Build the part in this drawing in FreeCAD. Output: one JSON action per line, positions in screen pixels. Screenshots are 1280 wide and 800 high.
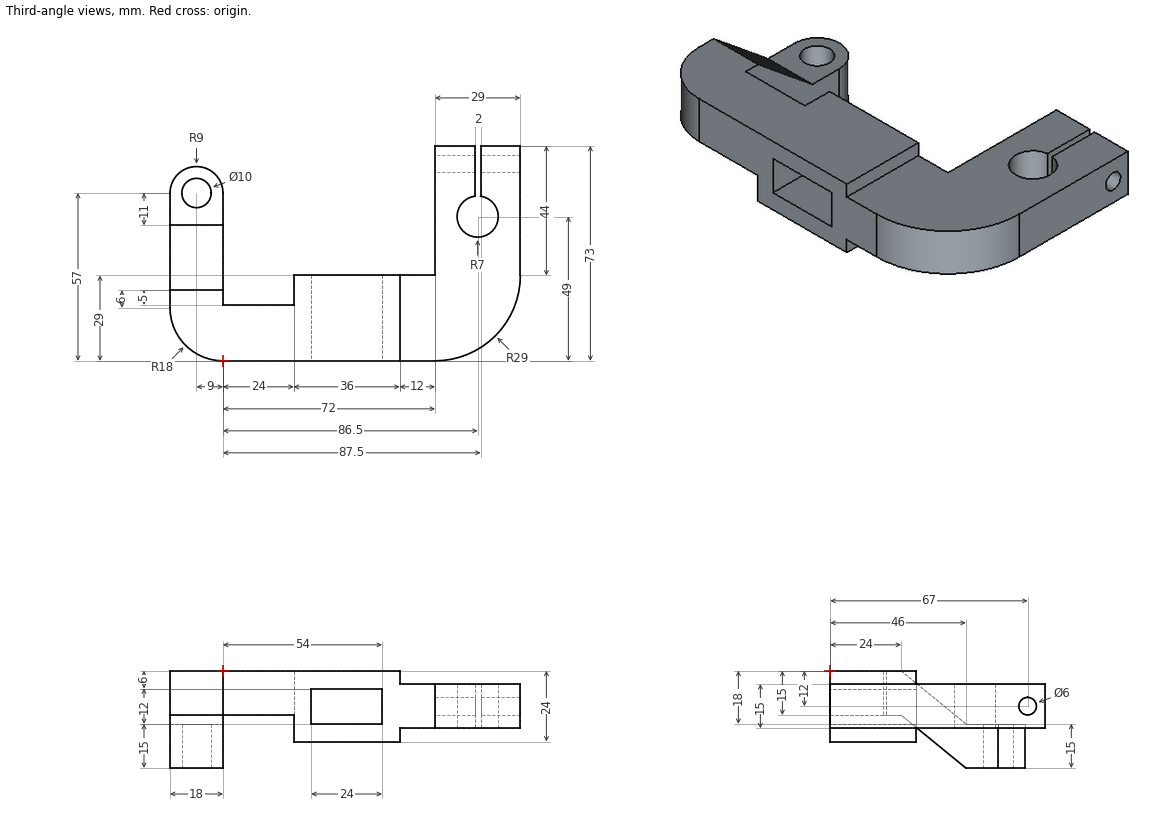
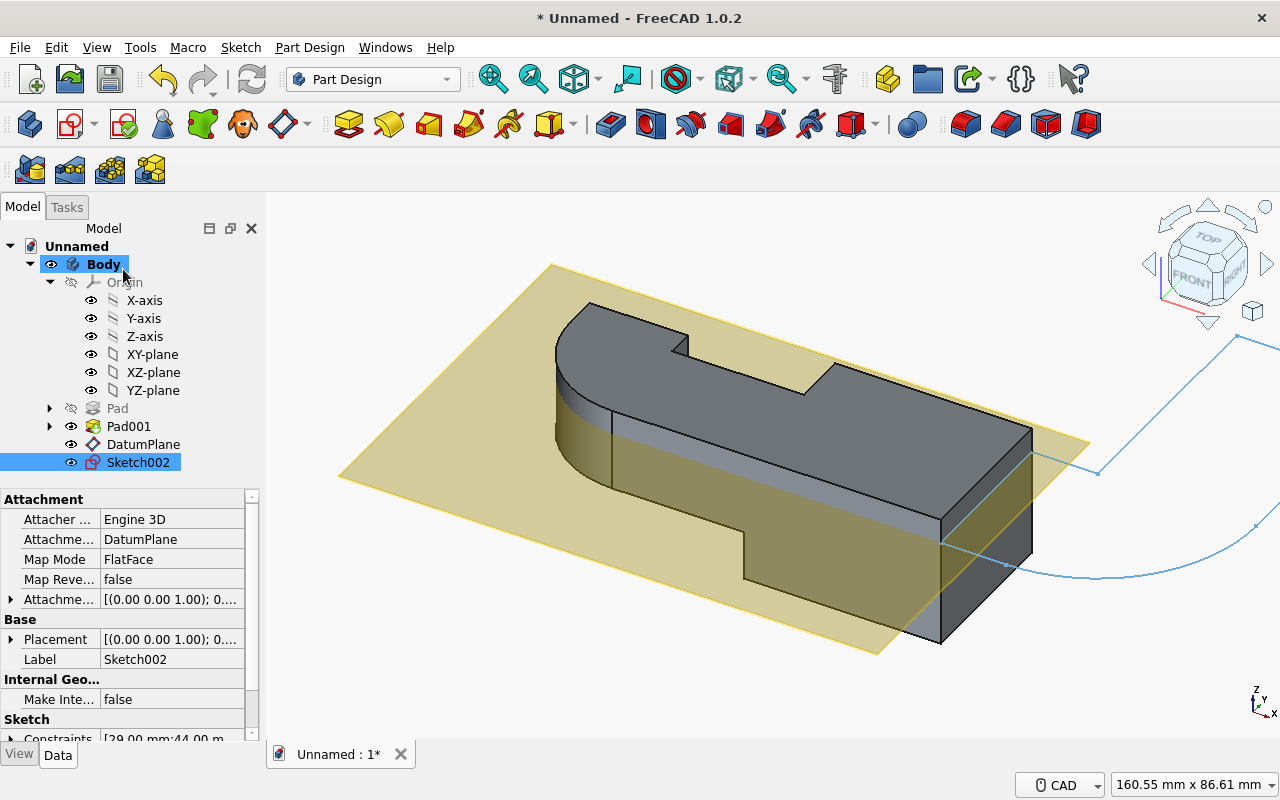
{"action": "left_click", "coordinate": [350, 124]}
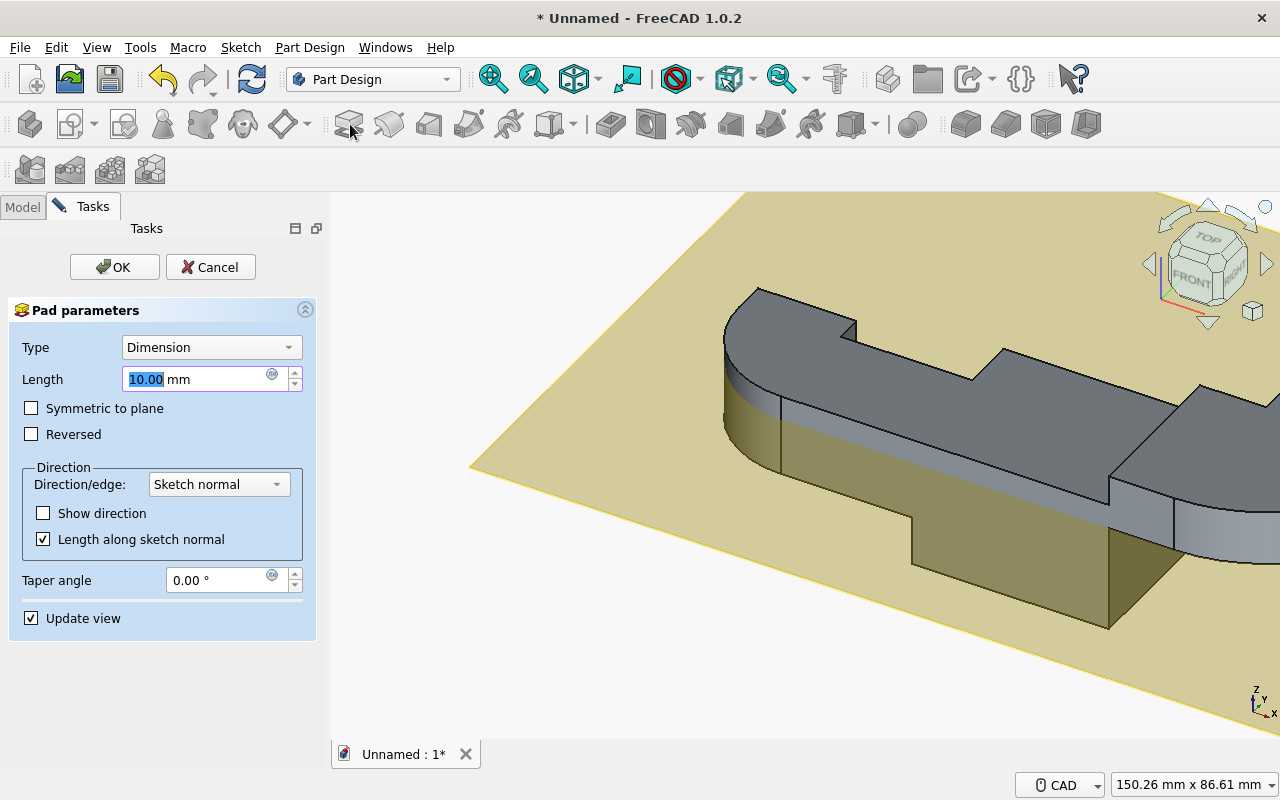
{"action": "type", "text": "15"}
{"action": "key", "text": "Tab"}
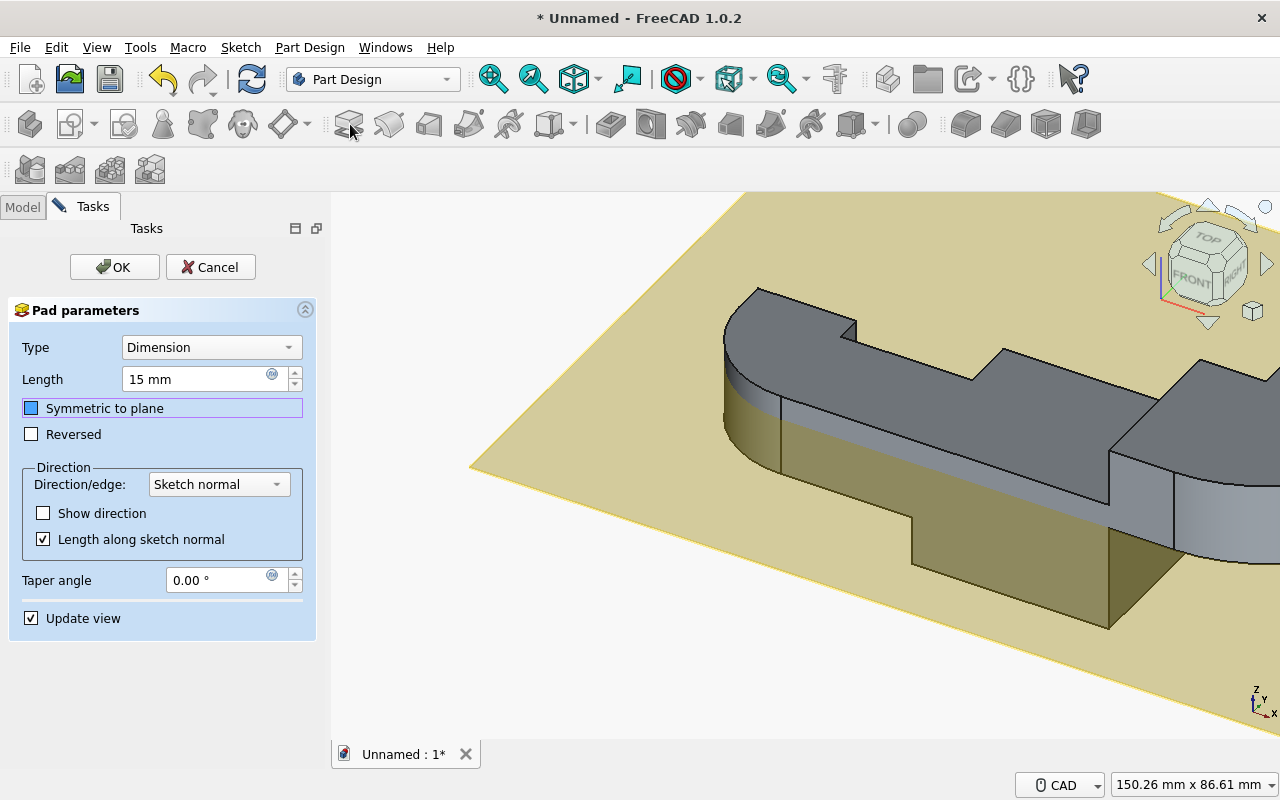
{"action": "left_click", "coordinate": [30, 434]}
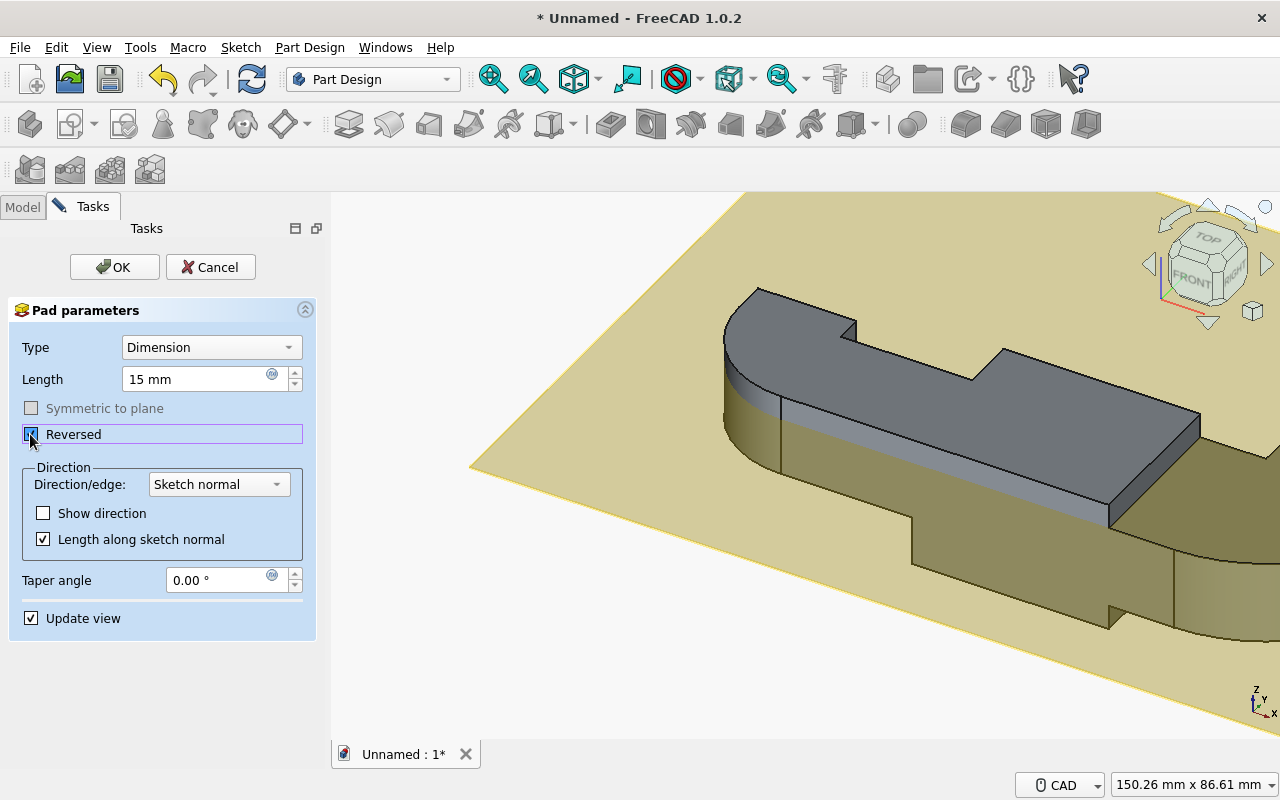
{"action": "left_click", "coordinate": [115, 267]}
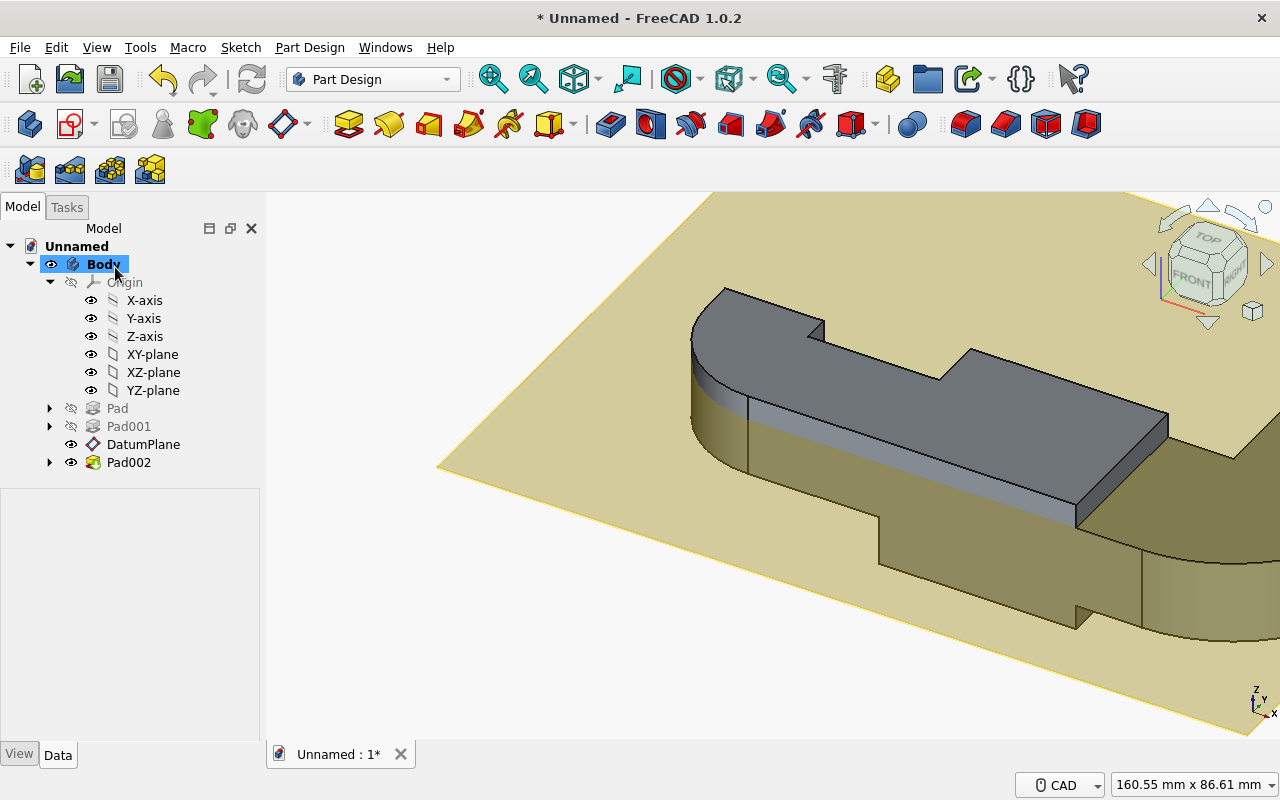
{"action": "left_click", "coordinate": [116, 444]}
{"action": "key", "text": "space"}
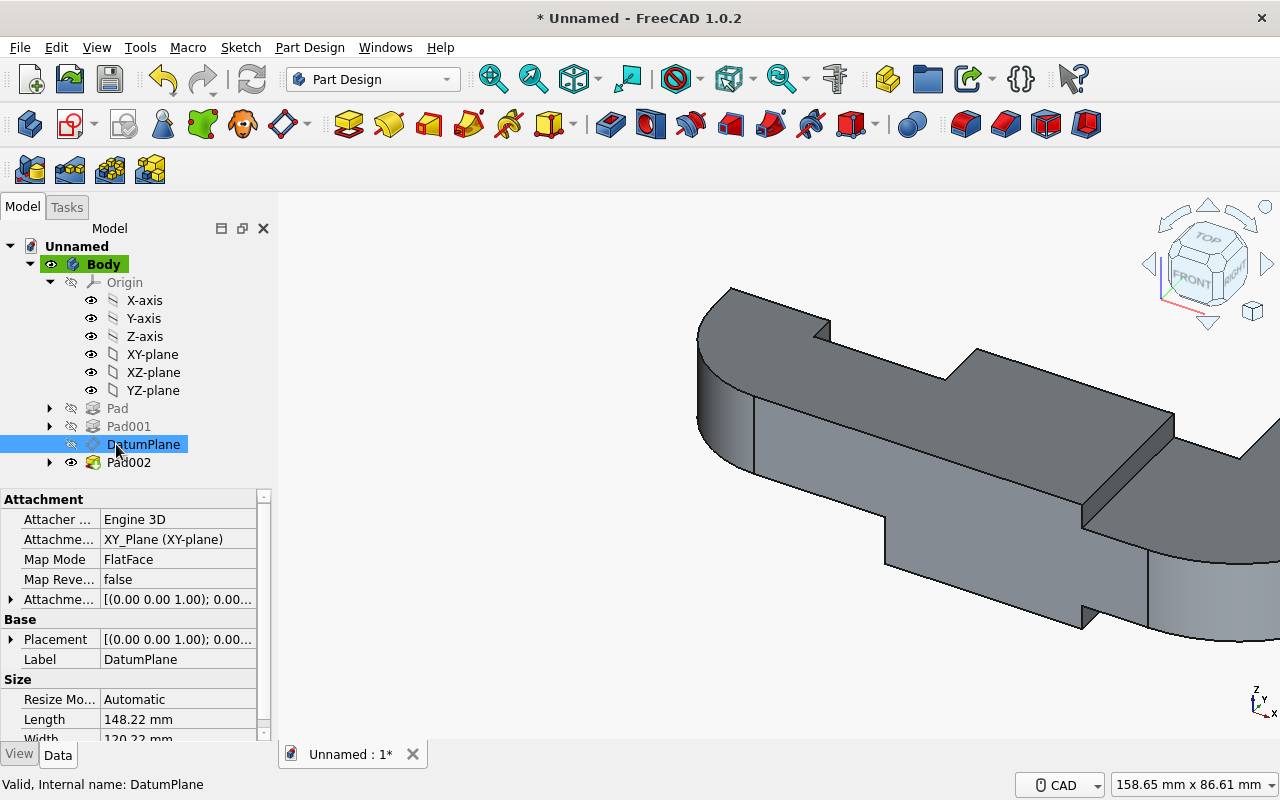
{"action": "key", "text": "v f"}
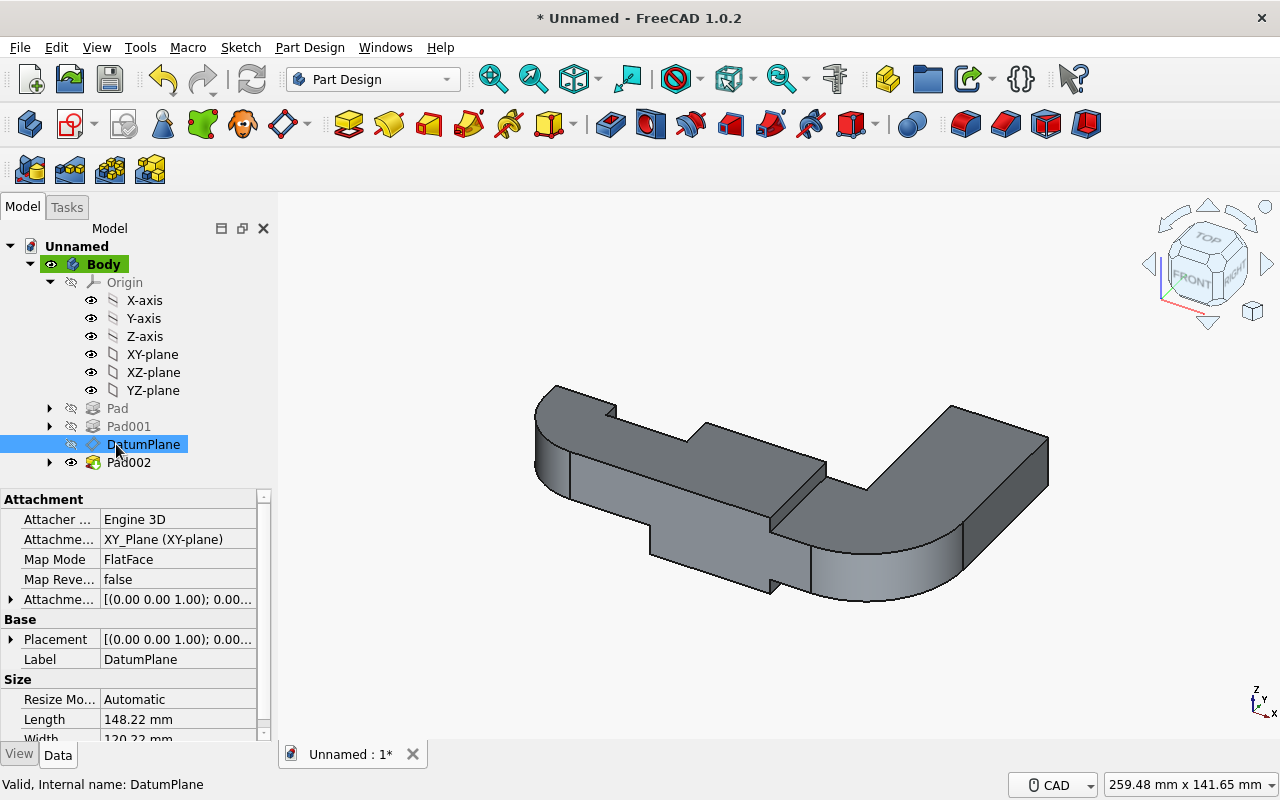
{"action": "key", "text": "6"}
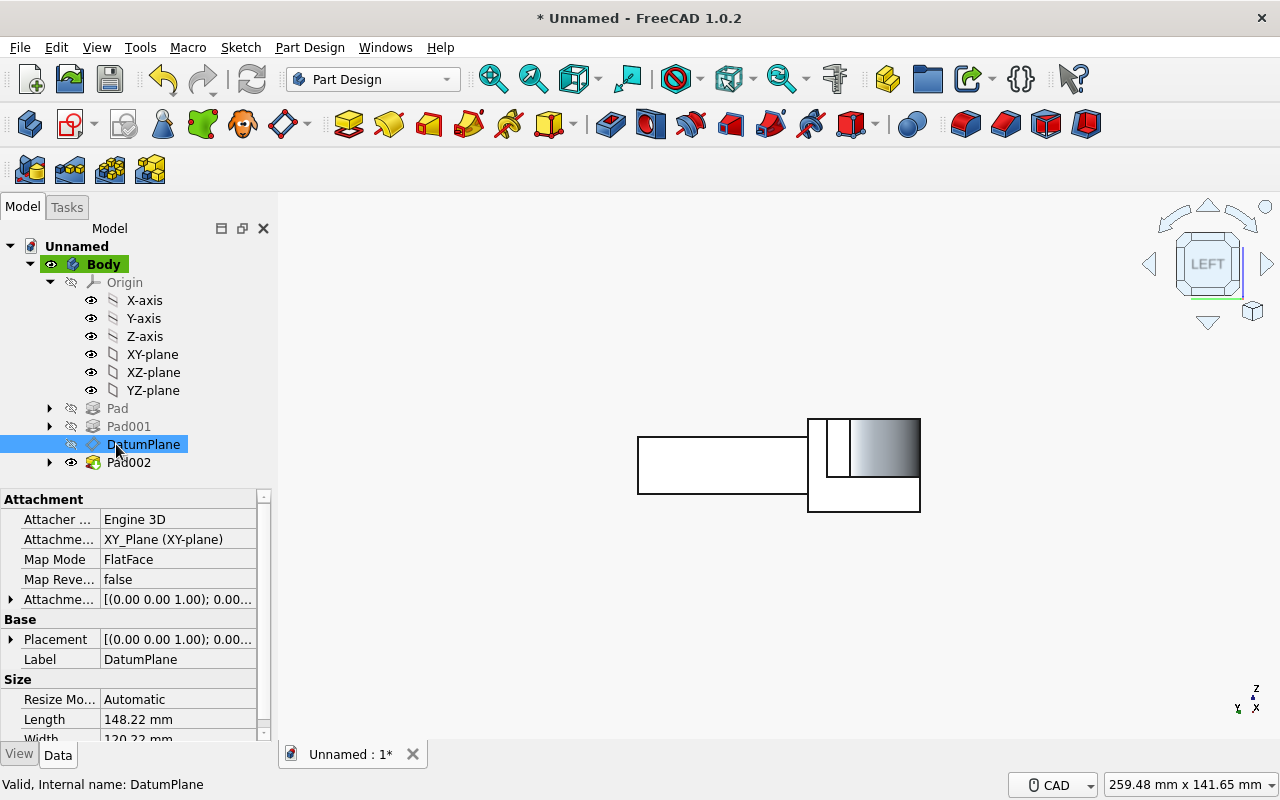
{"action": "left_click", "coordinate": [494, 80]}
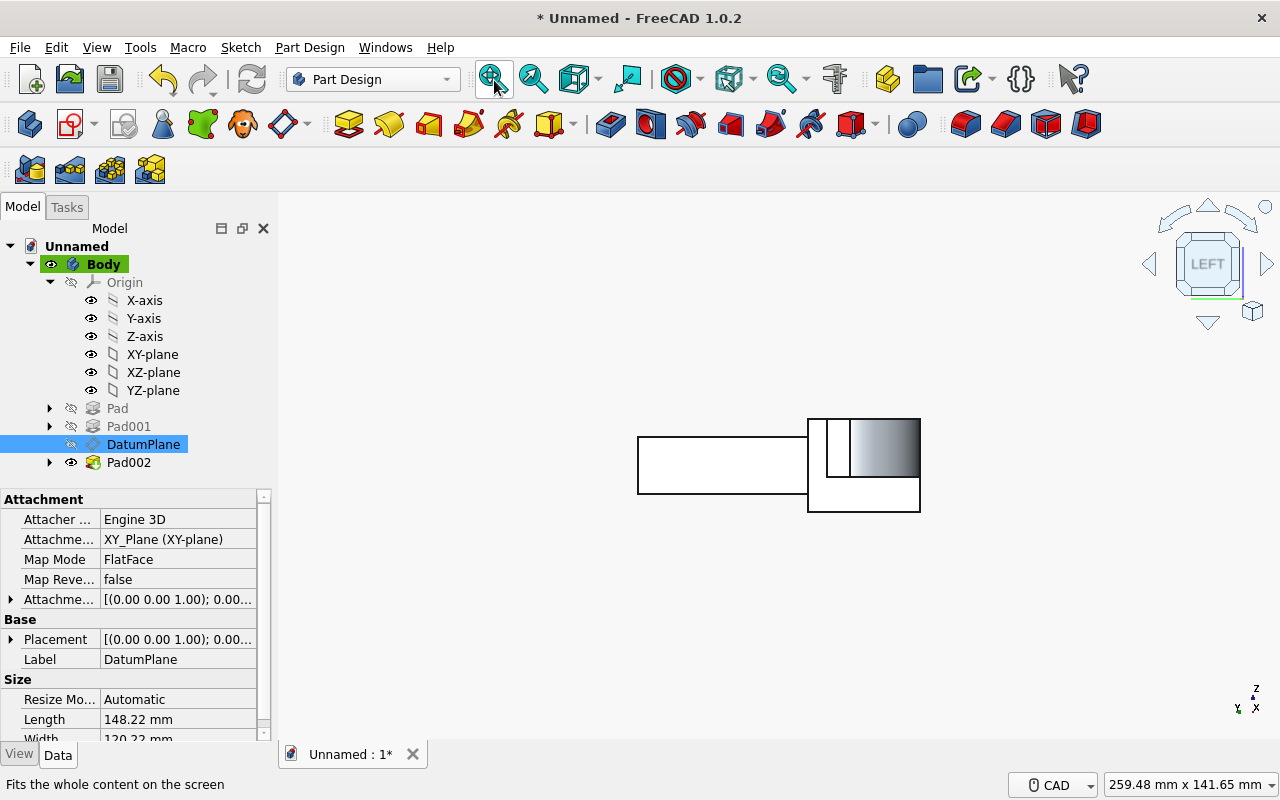
{"action": "left_click", "coordinate": [839, 431]}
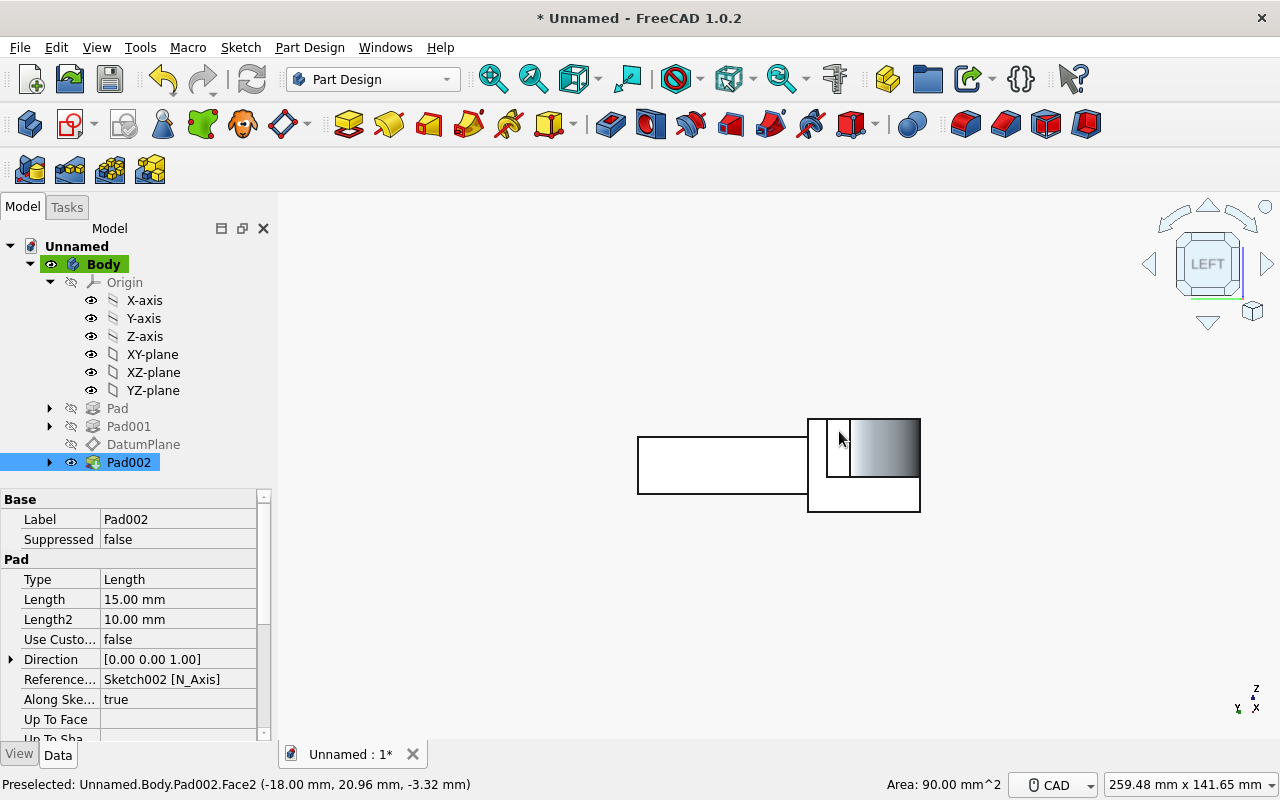
{"action": "left_click", "coordinate": [70, 124]}